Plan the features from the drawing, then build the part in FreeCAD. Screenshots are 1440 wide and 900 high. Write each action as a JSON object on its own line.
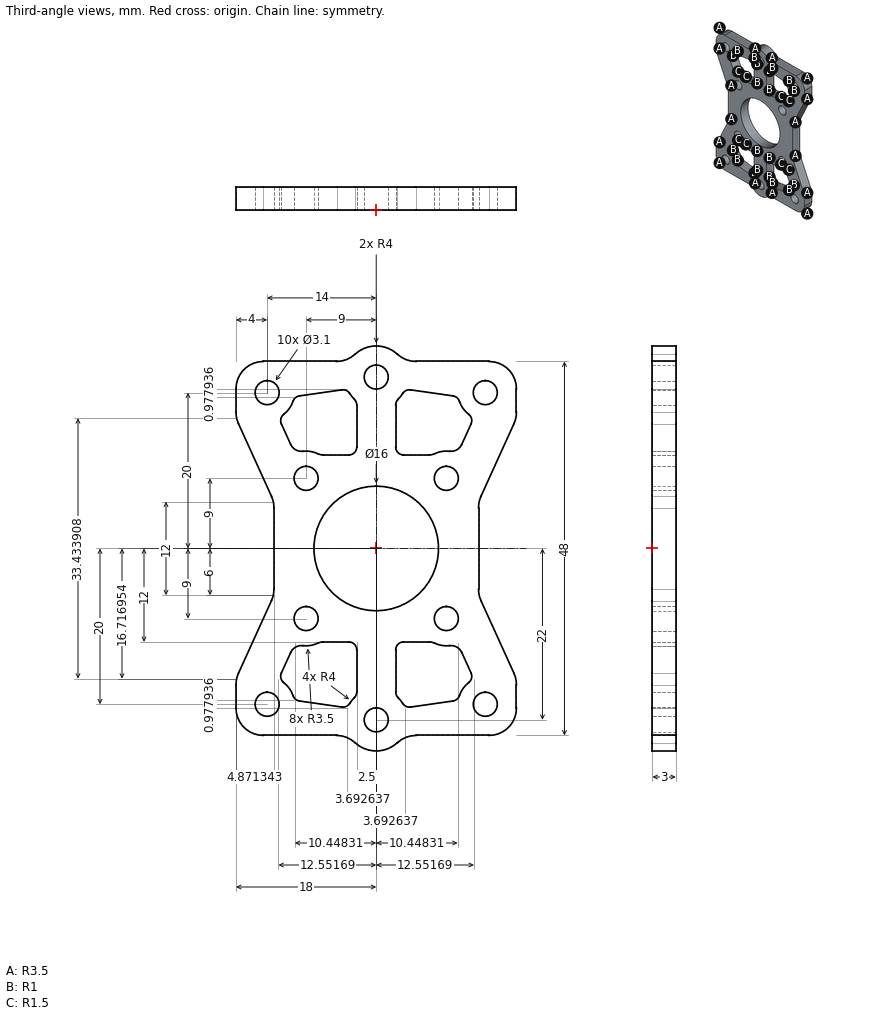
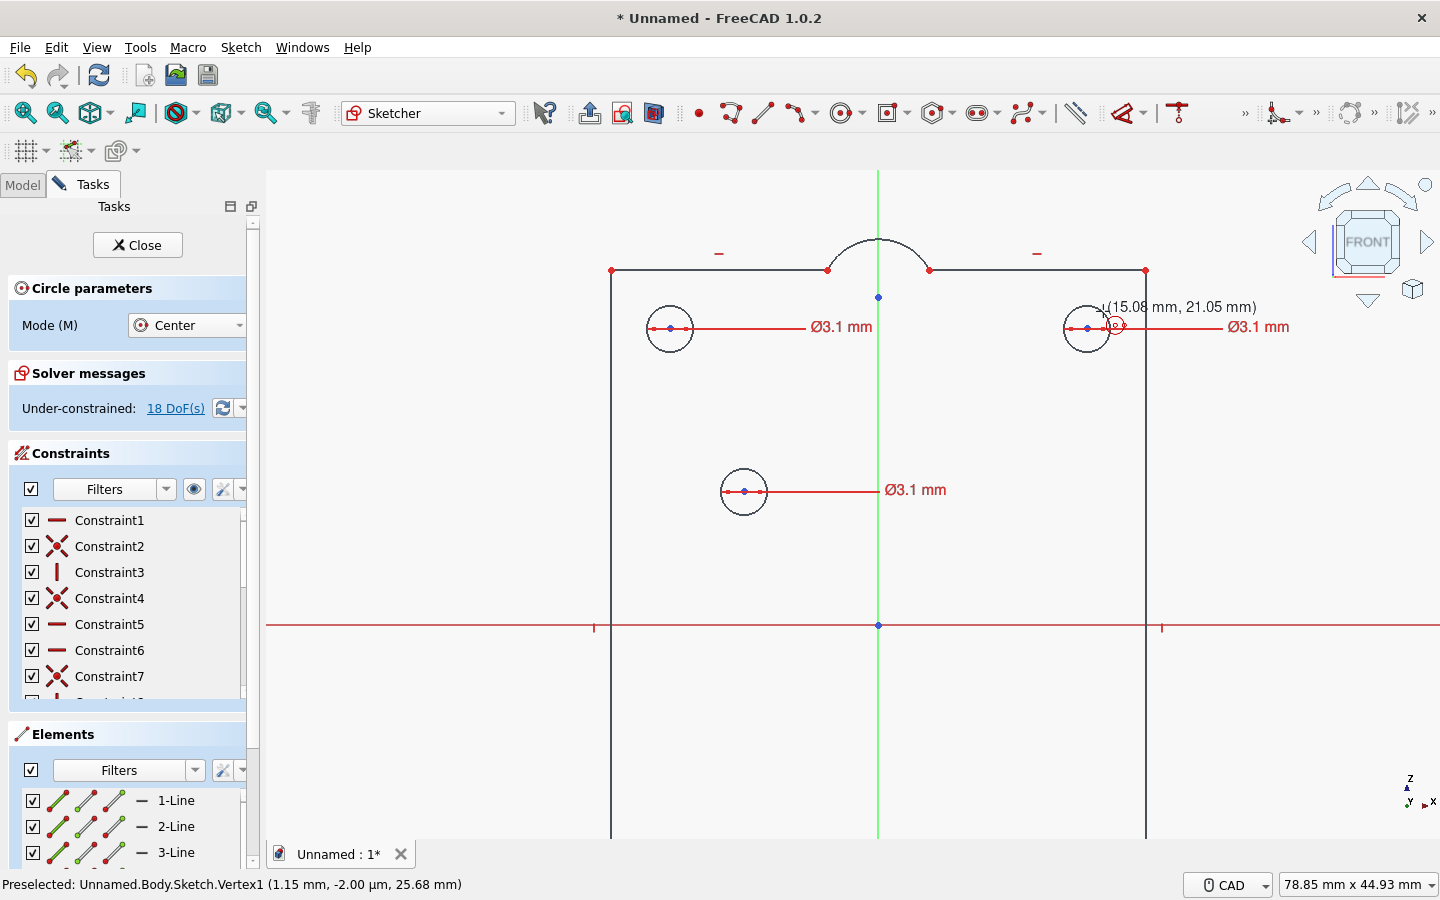
{"action": "left_click", "coordinate": [1012, 491]}
{"action": "mouse_move", "coordinate": [1029, 475]}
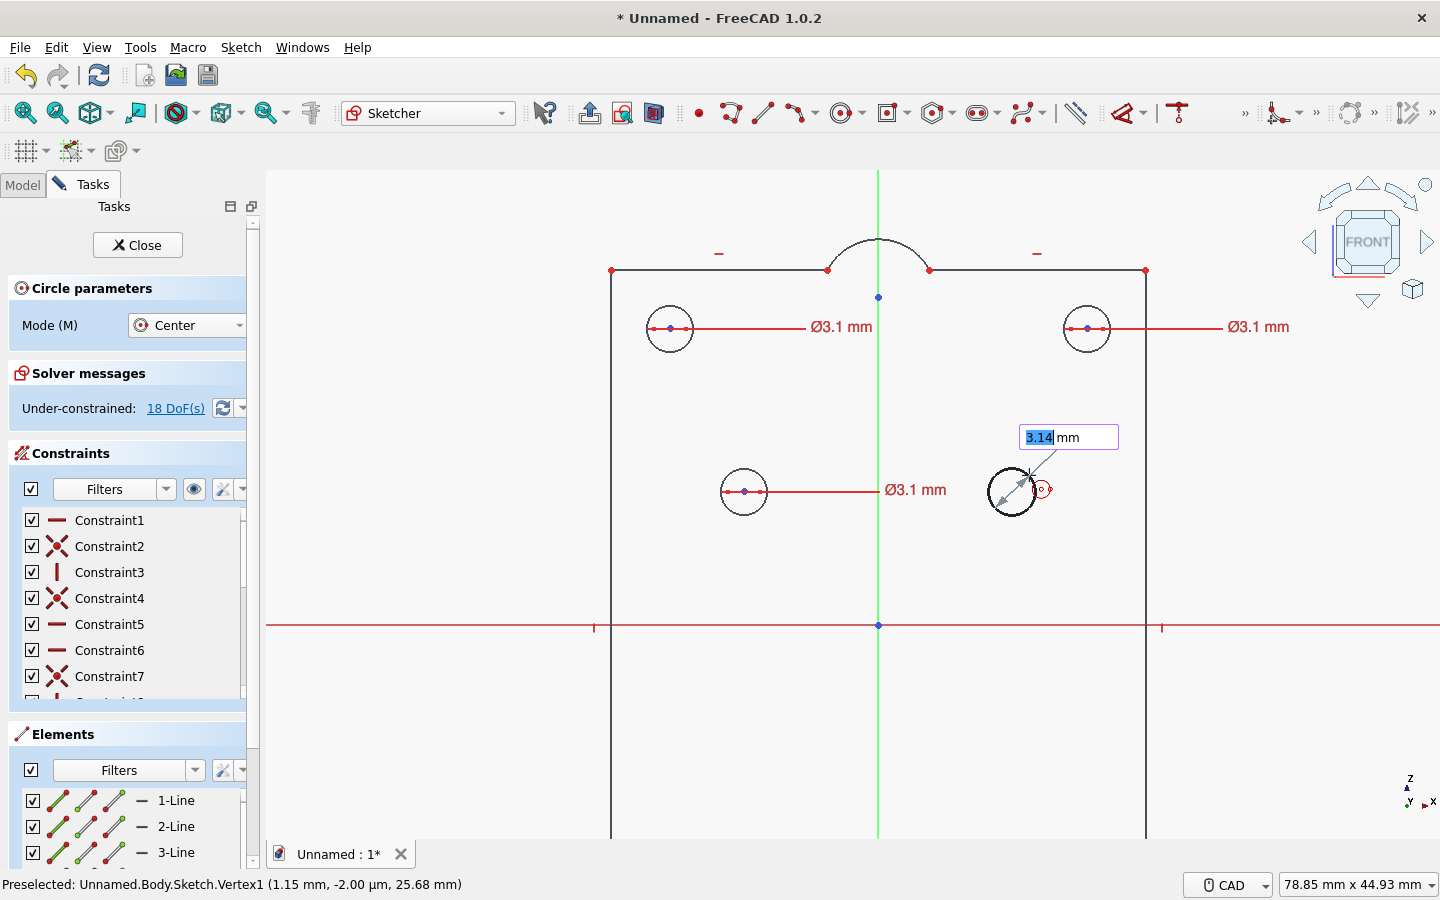
{"action": "type", "text": "3.1"}
{"action": "key", "text": "Return"}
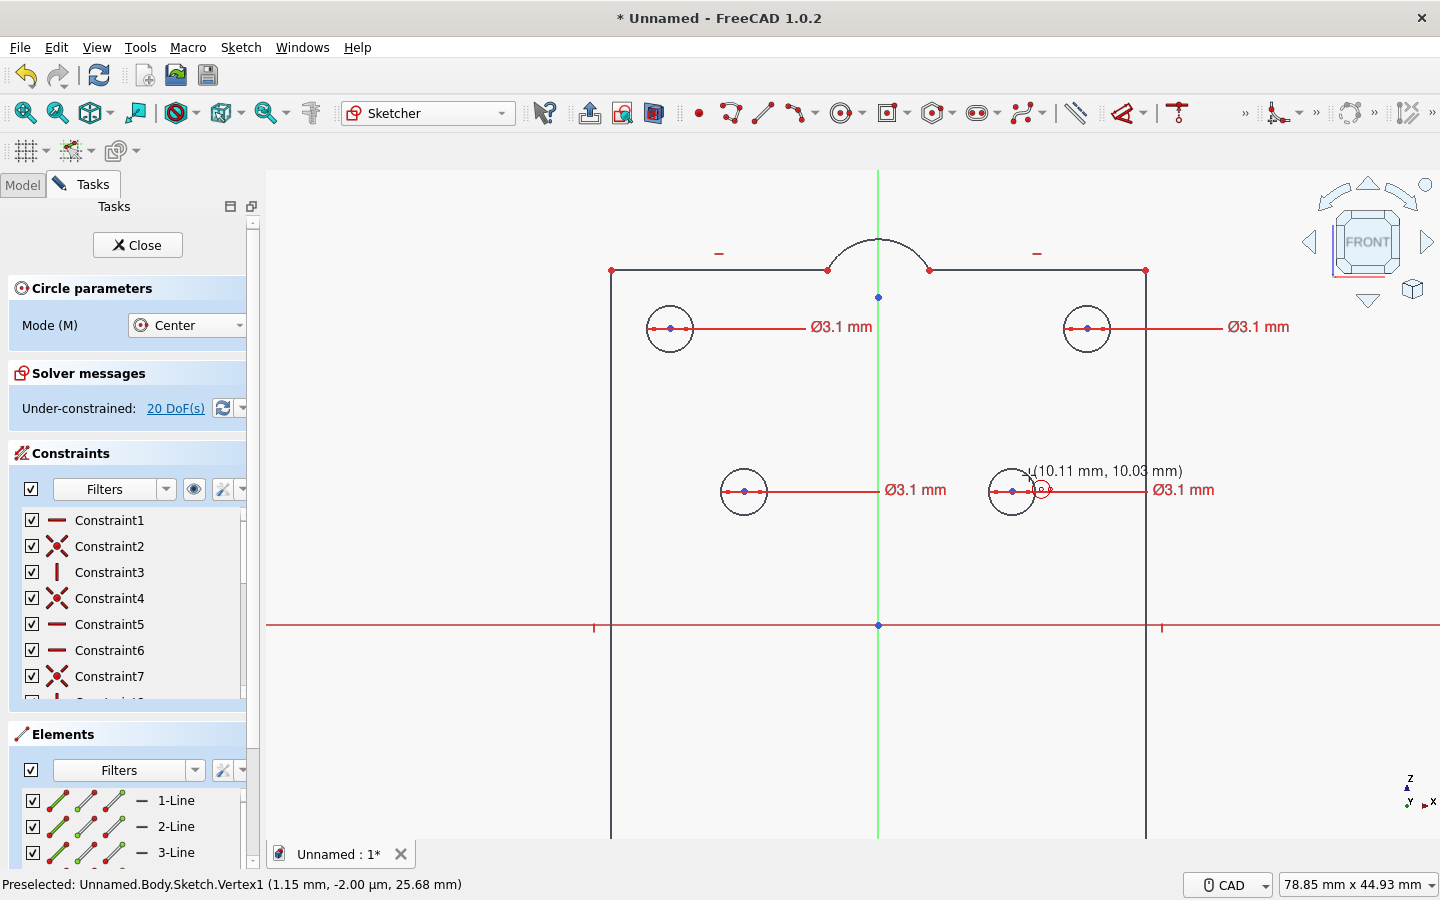
{"action": "left_click", "coordinate": [744, 759]}
{"action": "mouse_move", "coordinate": [761, 743]}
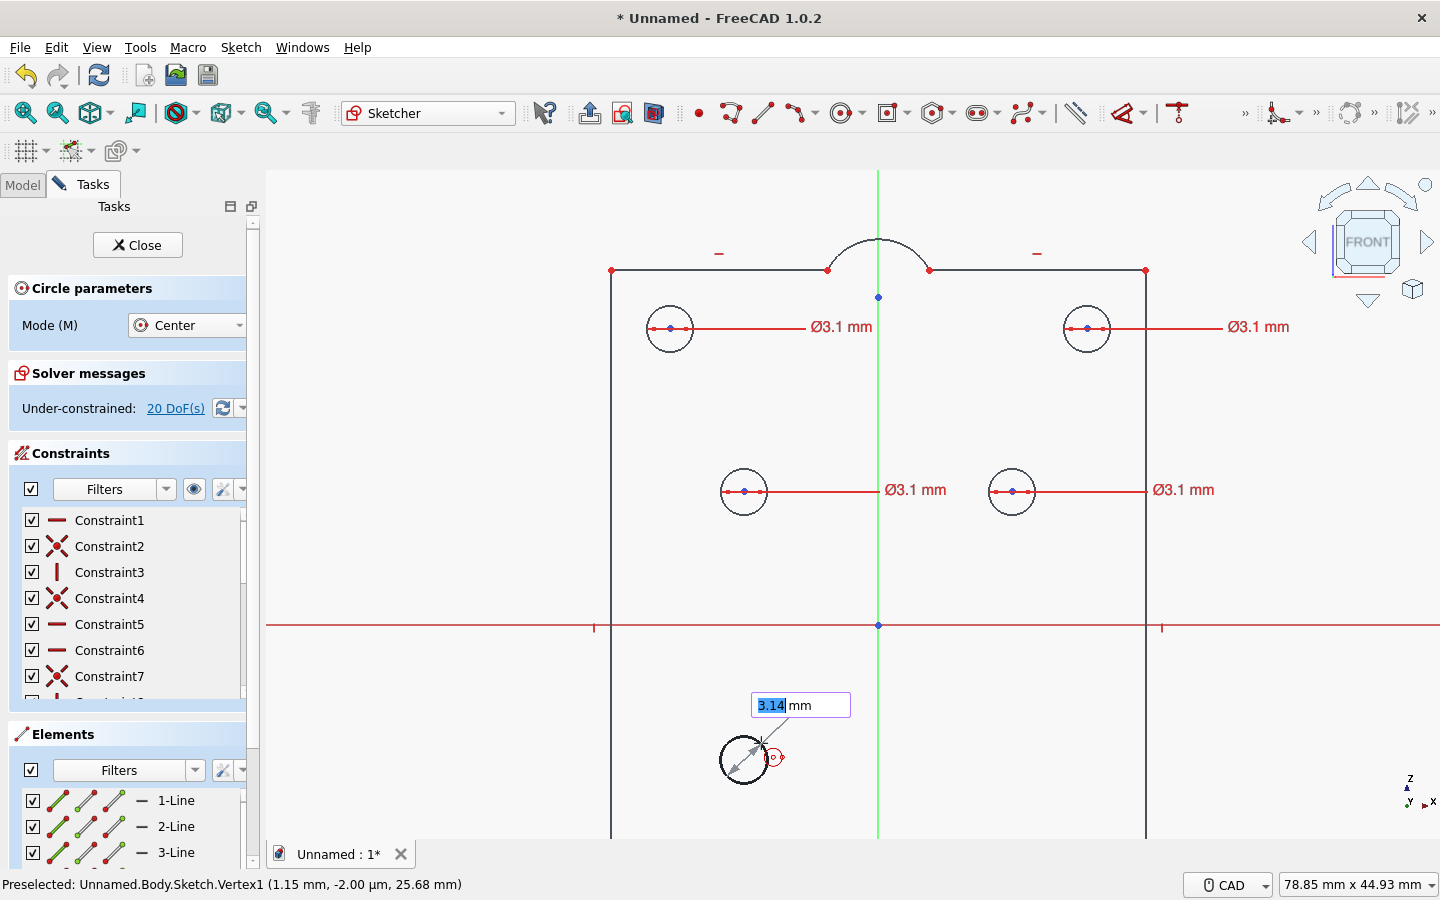
{"action": "type", "text": "3.1"}
{"action": "key", "text": "Return"}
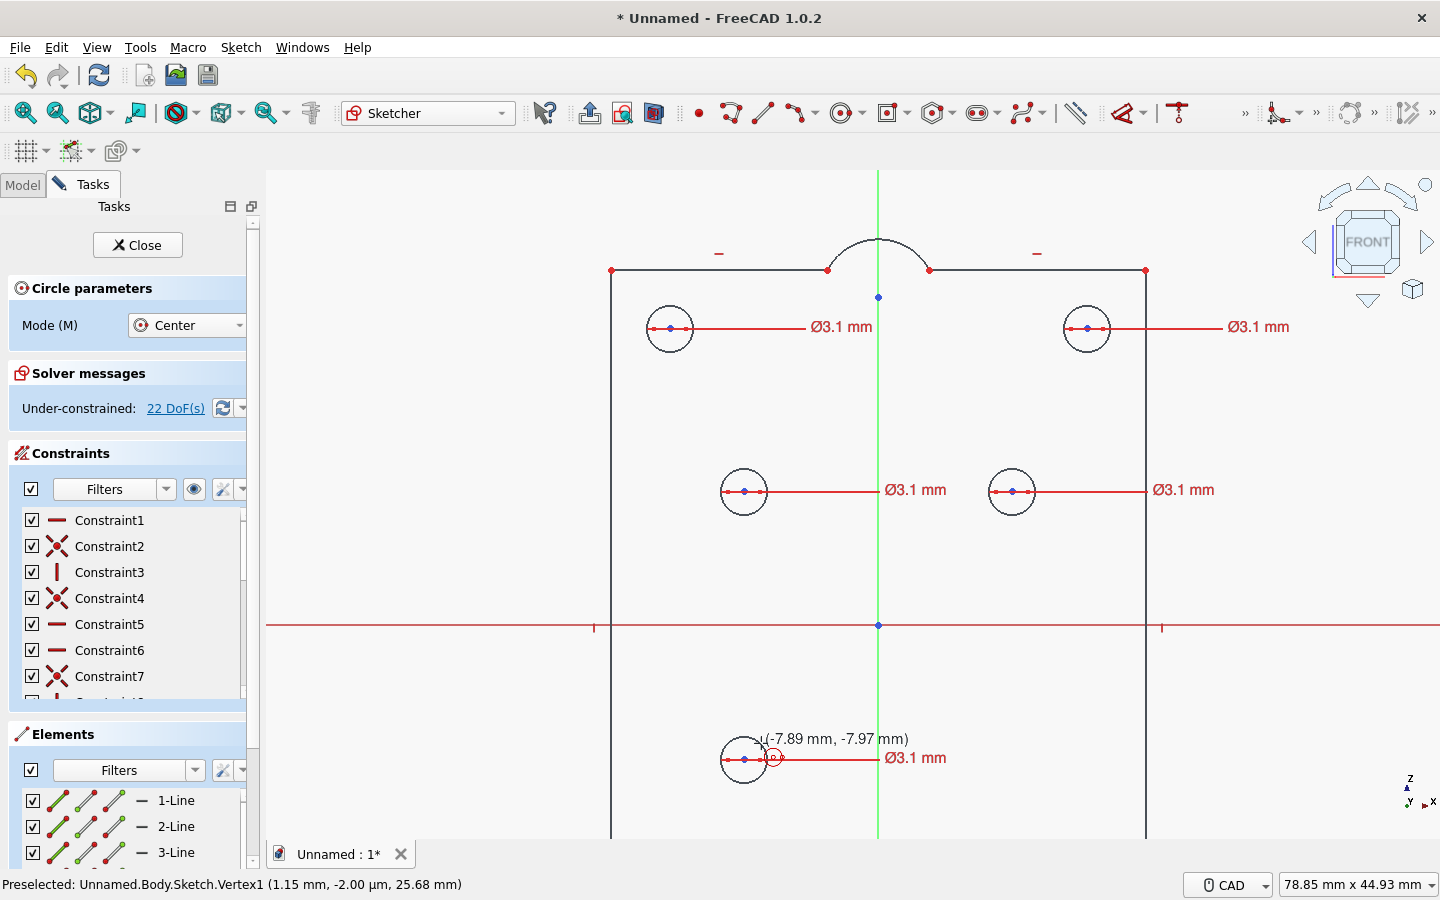
{"action": "scroll", "coordinate": [670, 357], "scroll_direction": "down", "scroll_amount": 3}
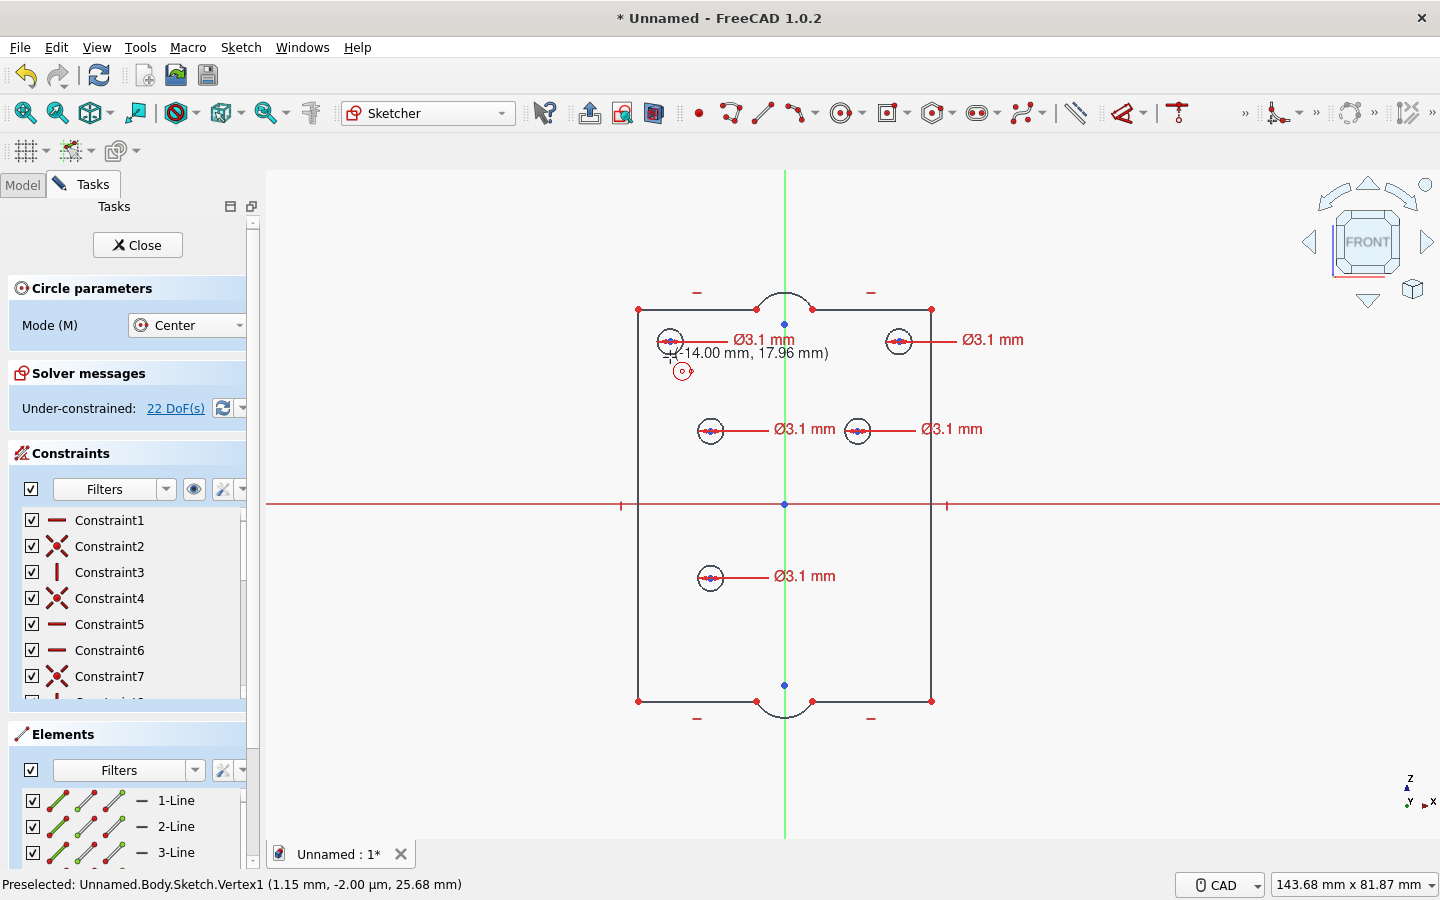
{"action": "scroll", "coordinate": [670, 668], "scroll_direction": "up", "scroll_amount": 3}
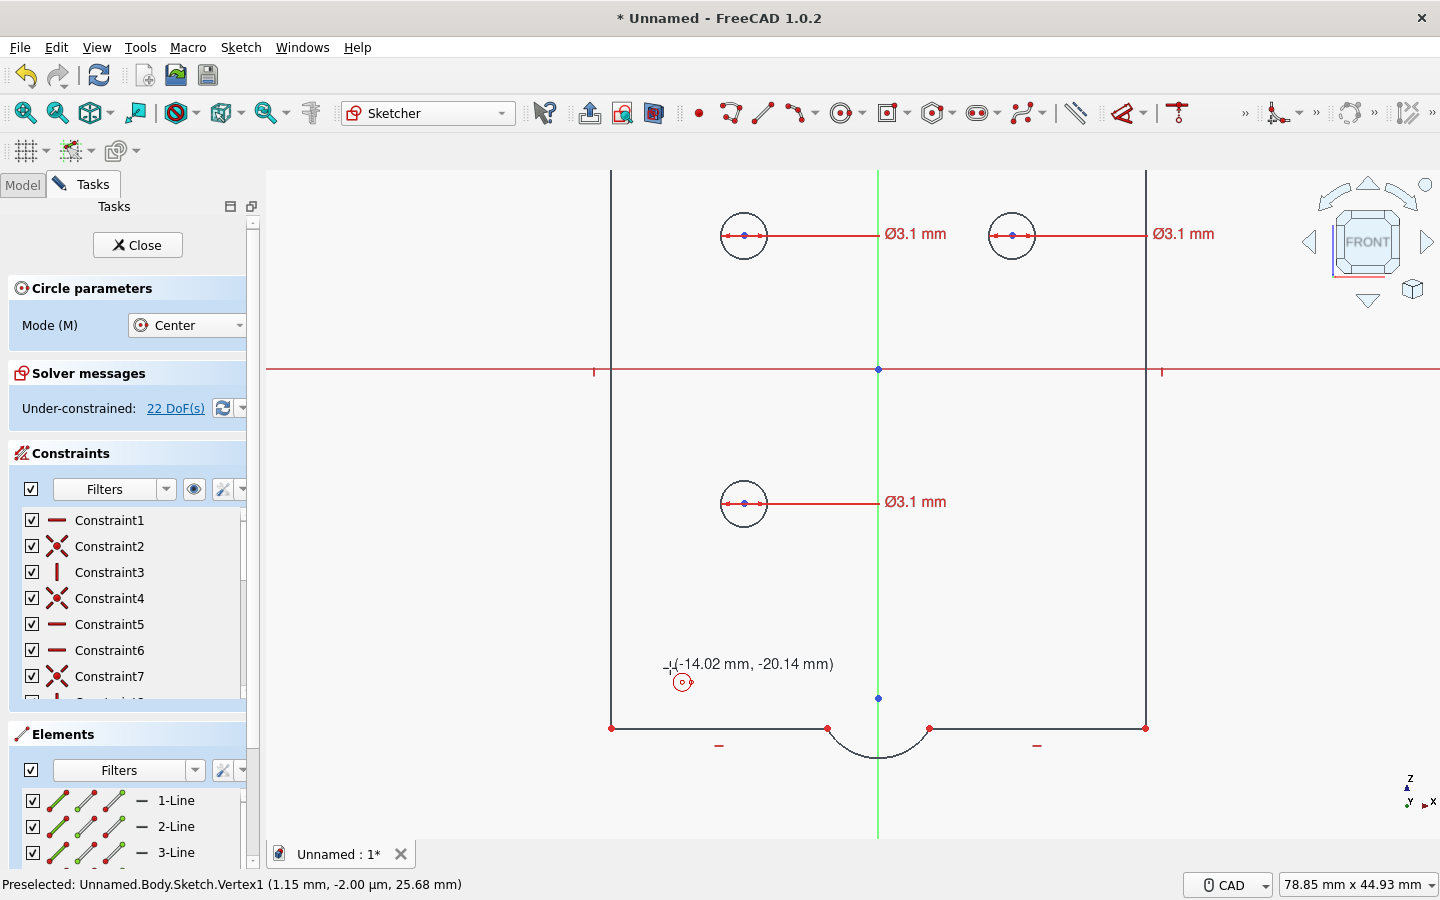
{"action": "left_click", "coordinate": [670, 667]}
{"action": "mouse_move", "coordinate": [686, 651]}